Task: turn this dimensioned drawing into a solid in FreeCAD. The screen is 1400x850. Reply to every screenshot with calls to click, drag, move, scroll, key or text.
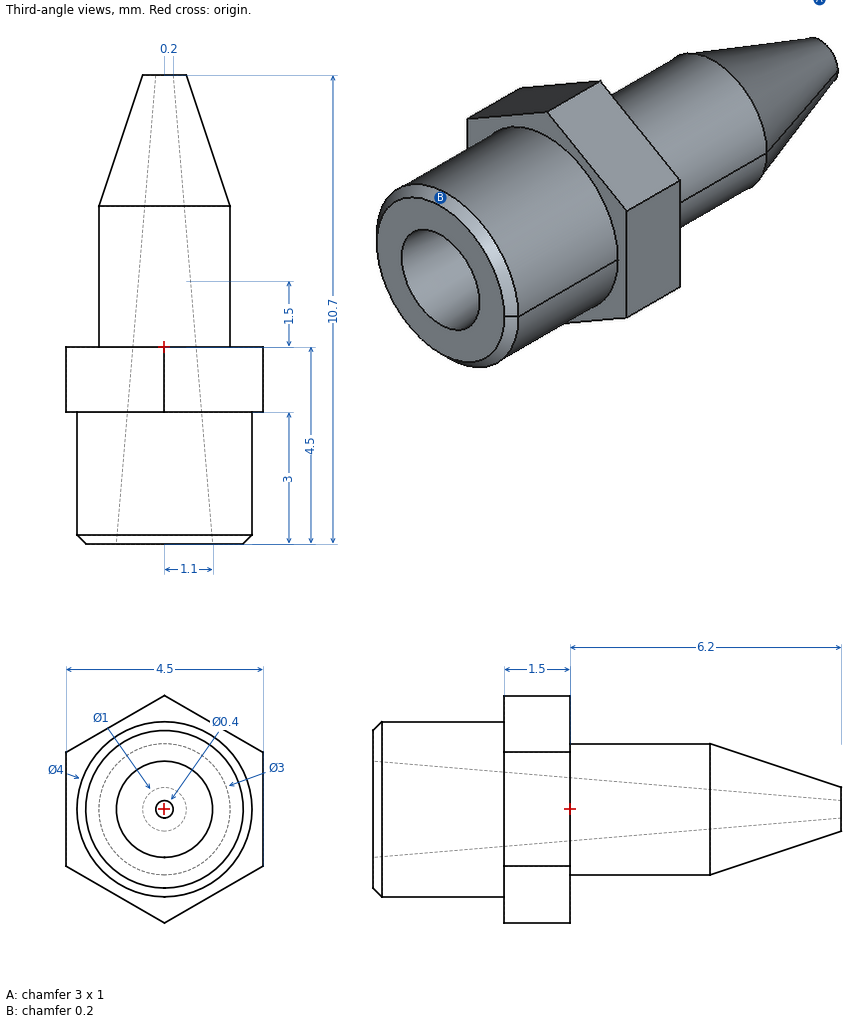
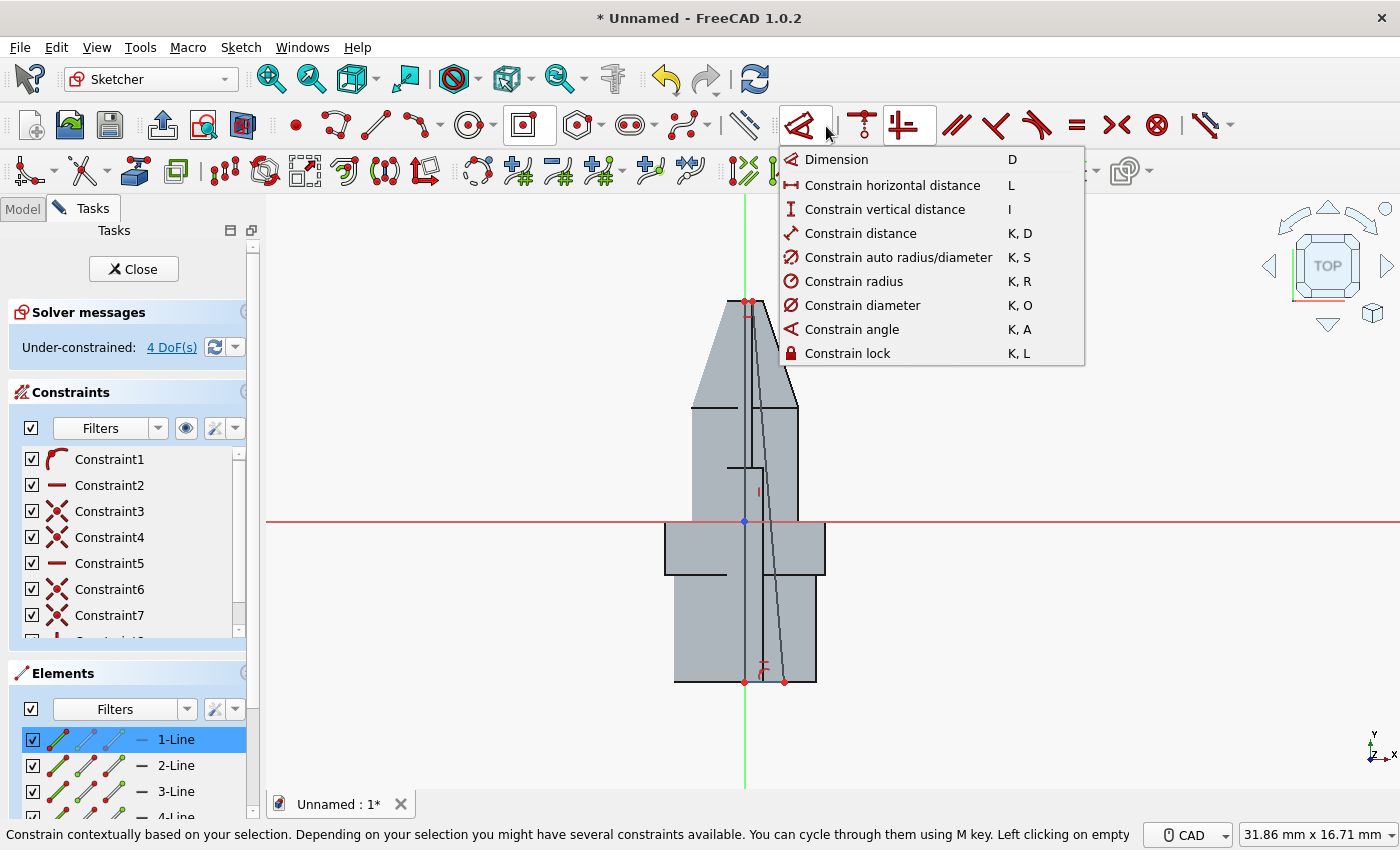
click(932, 185)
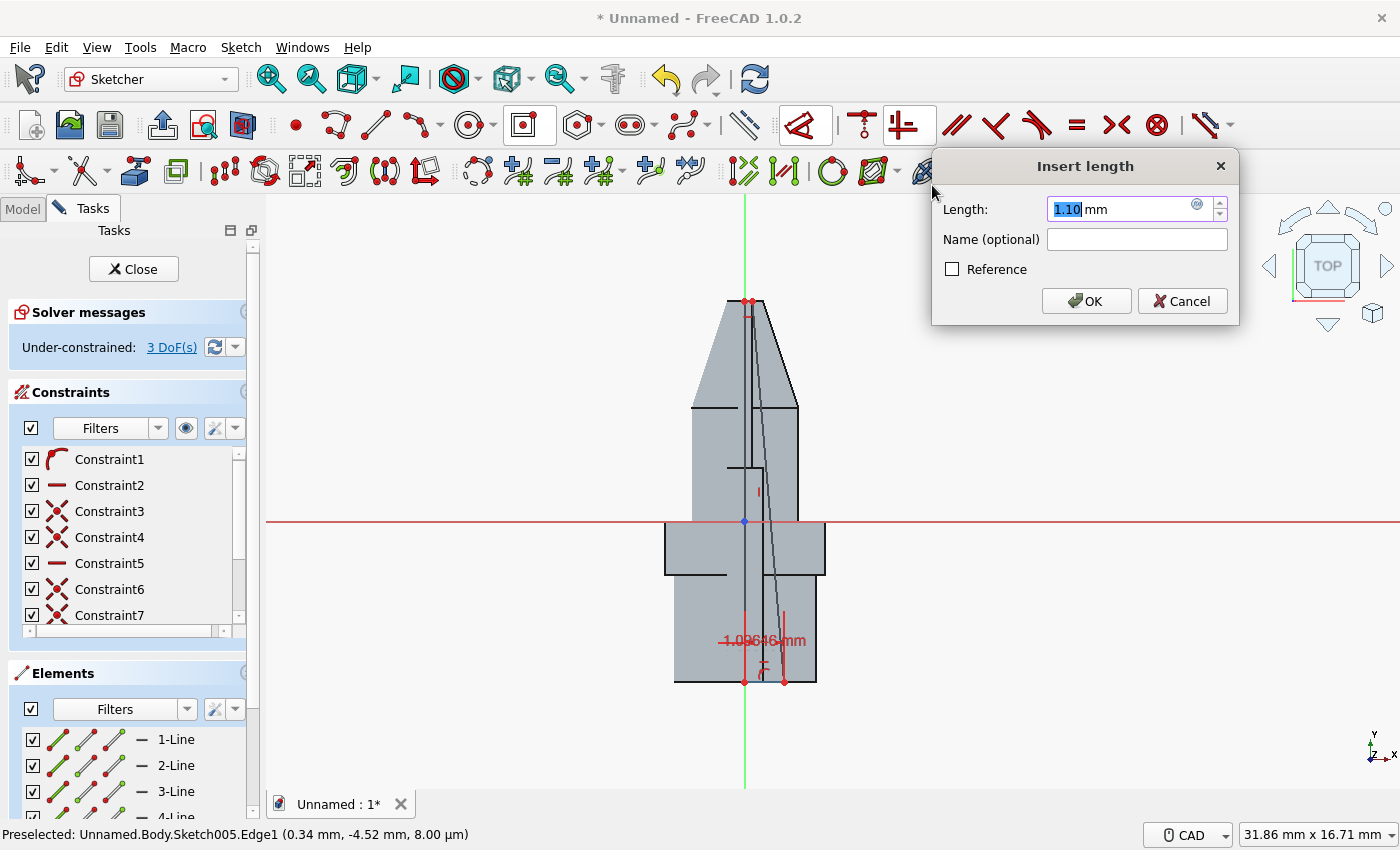
text(1.1)
key(Return)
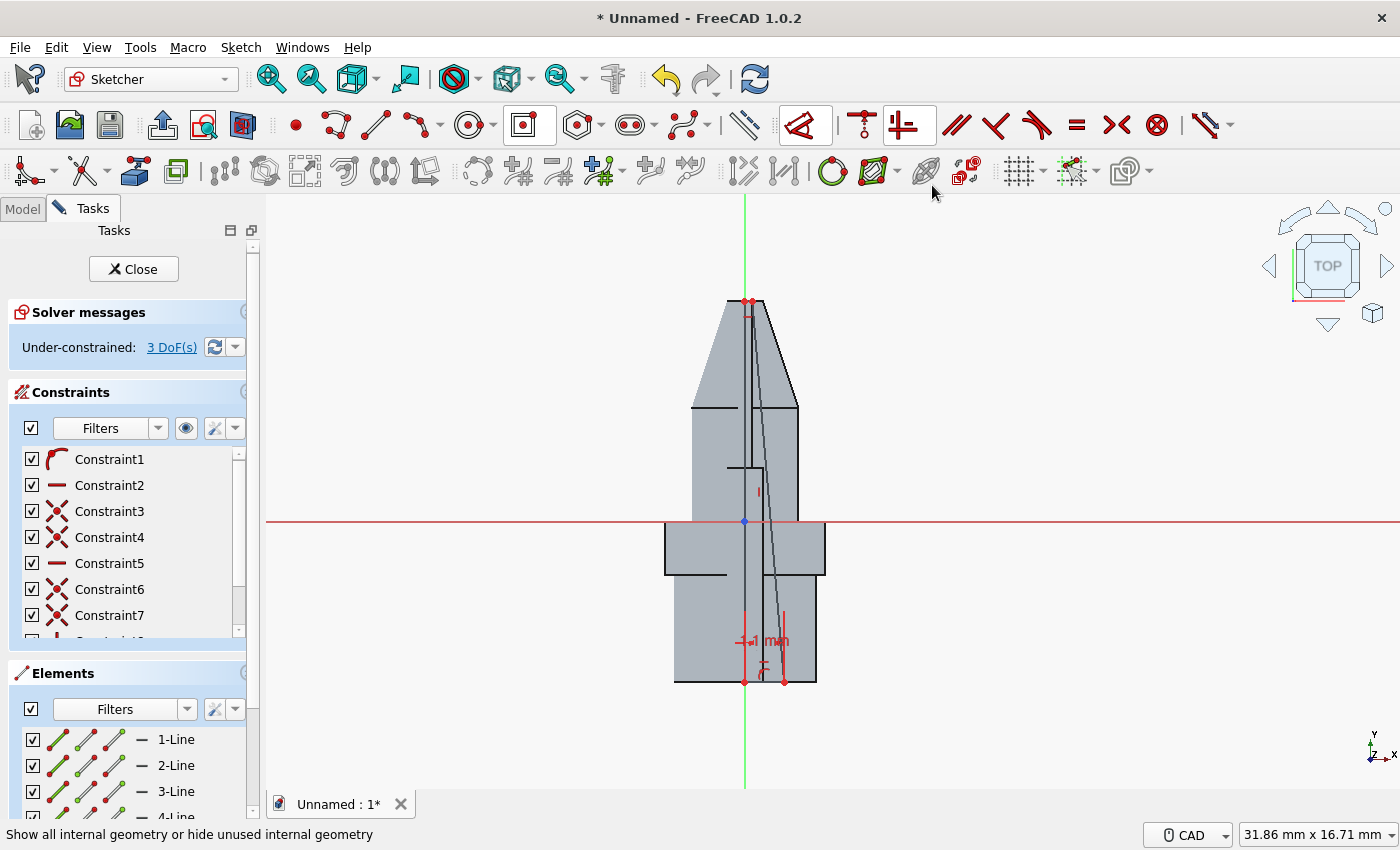
scroll(749, 301, up, 9)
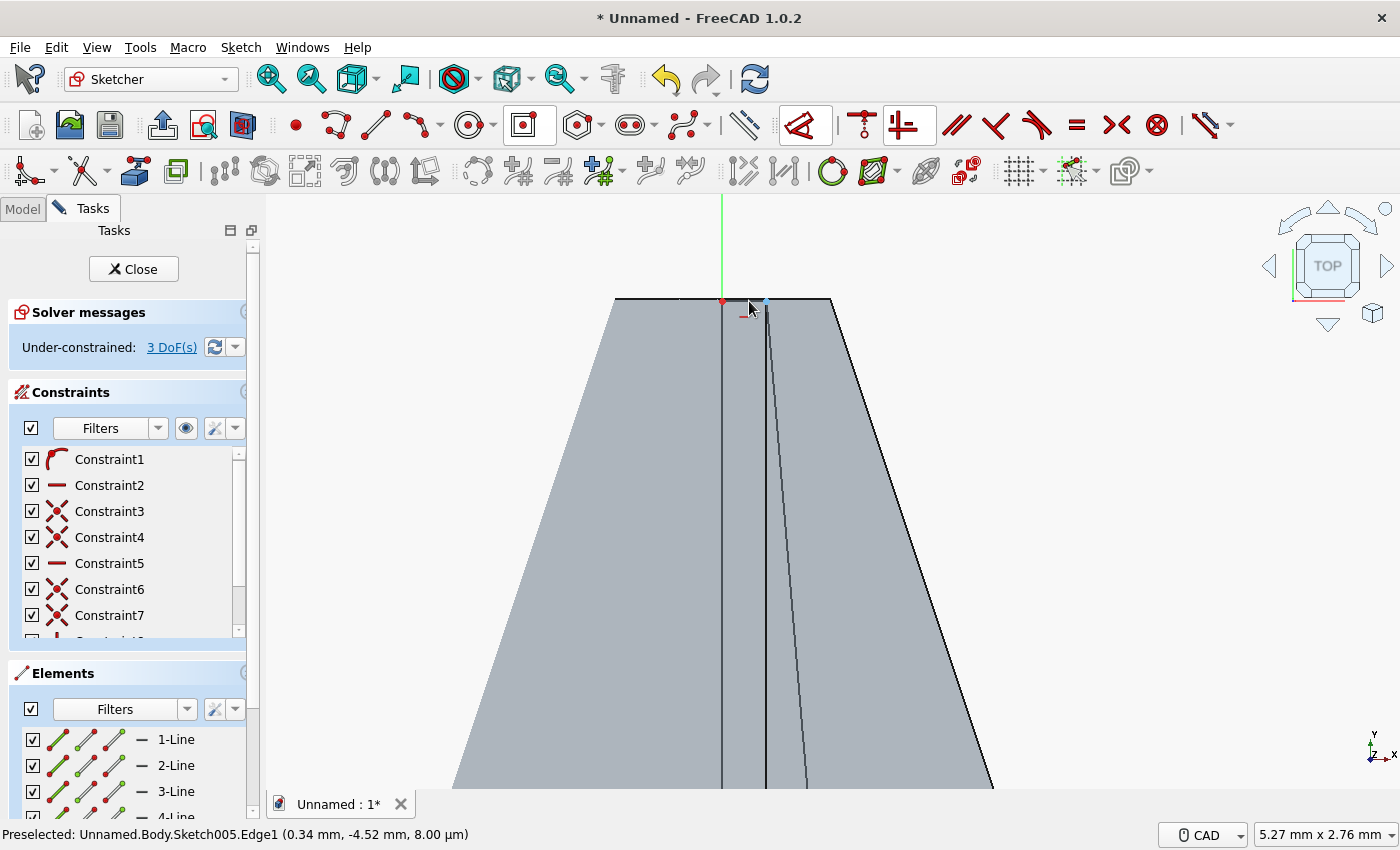
click(745, 301)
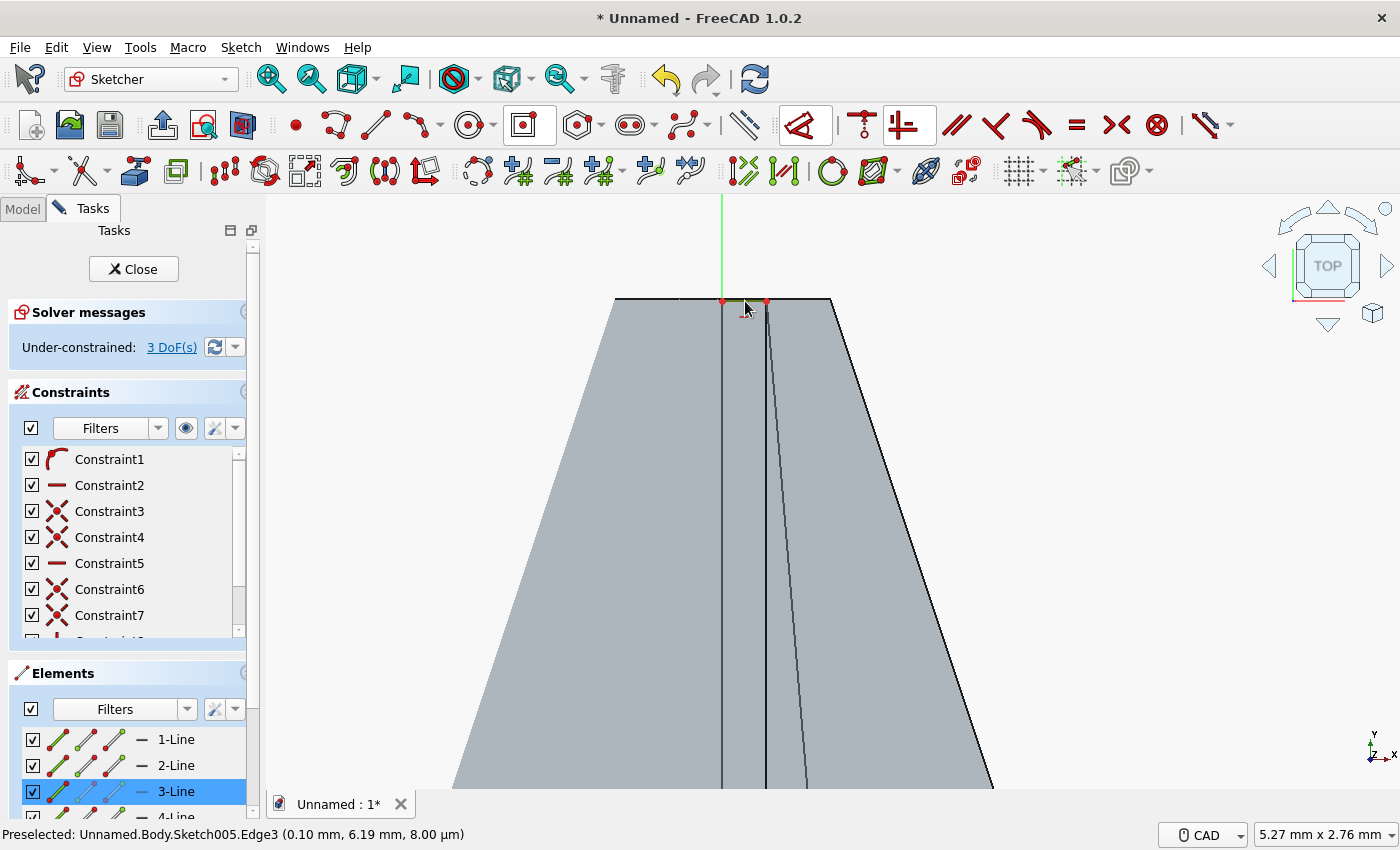
click(826, 126)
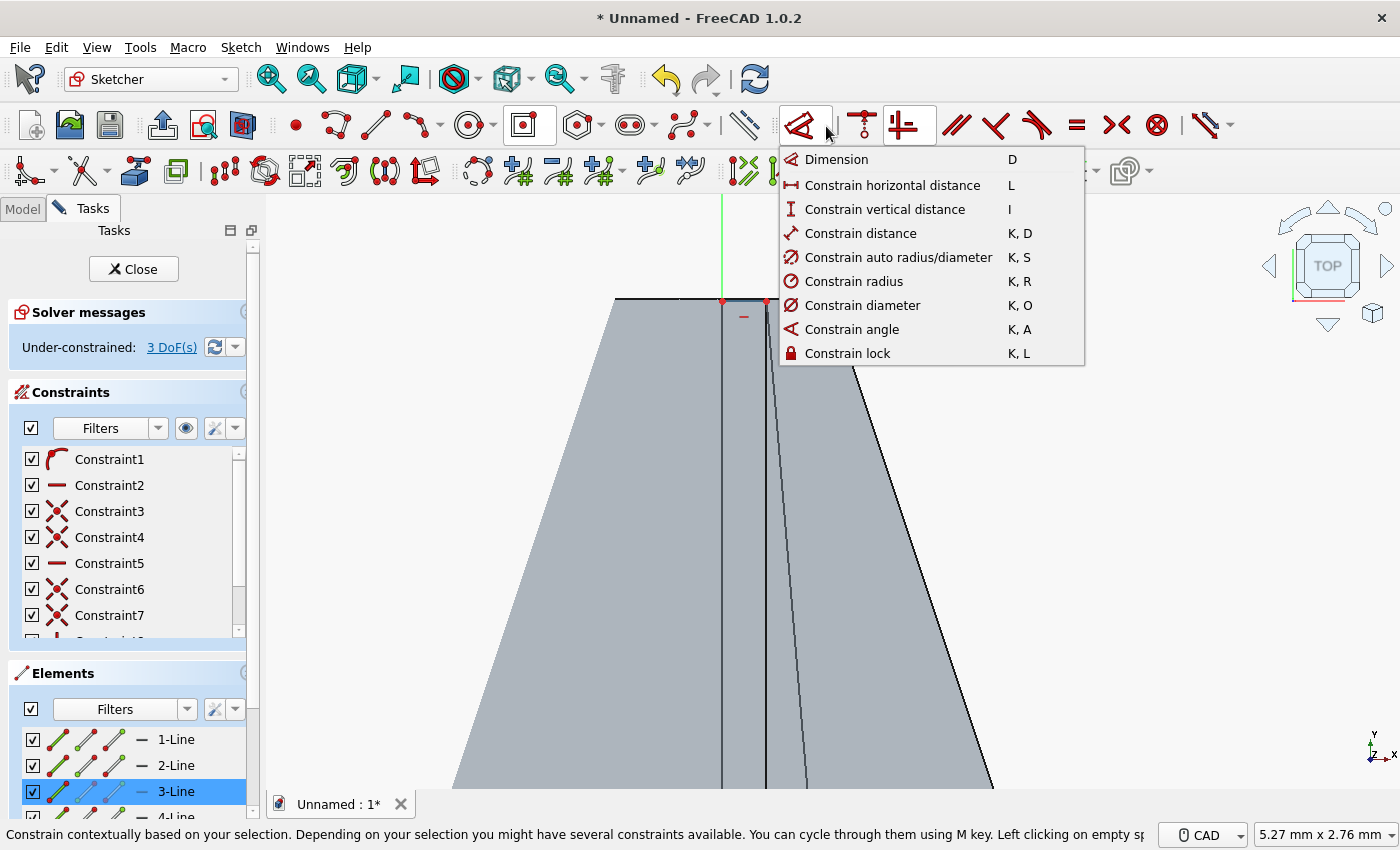
click(932, 185)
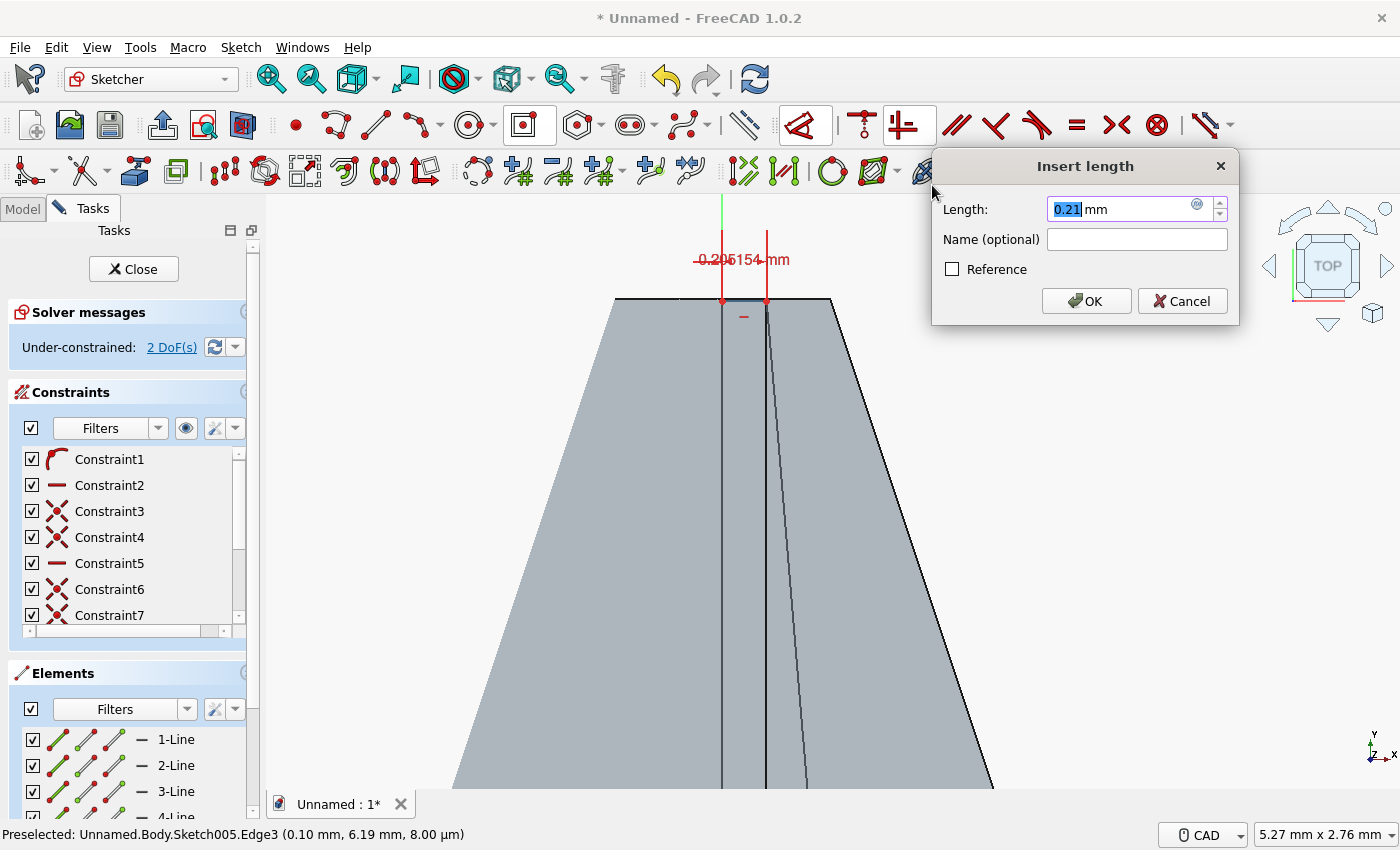
text(0.2)
key(Return)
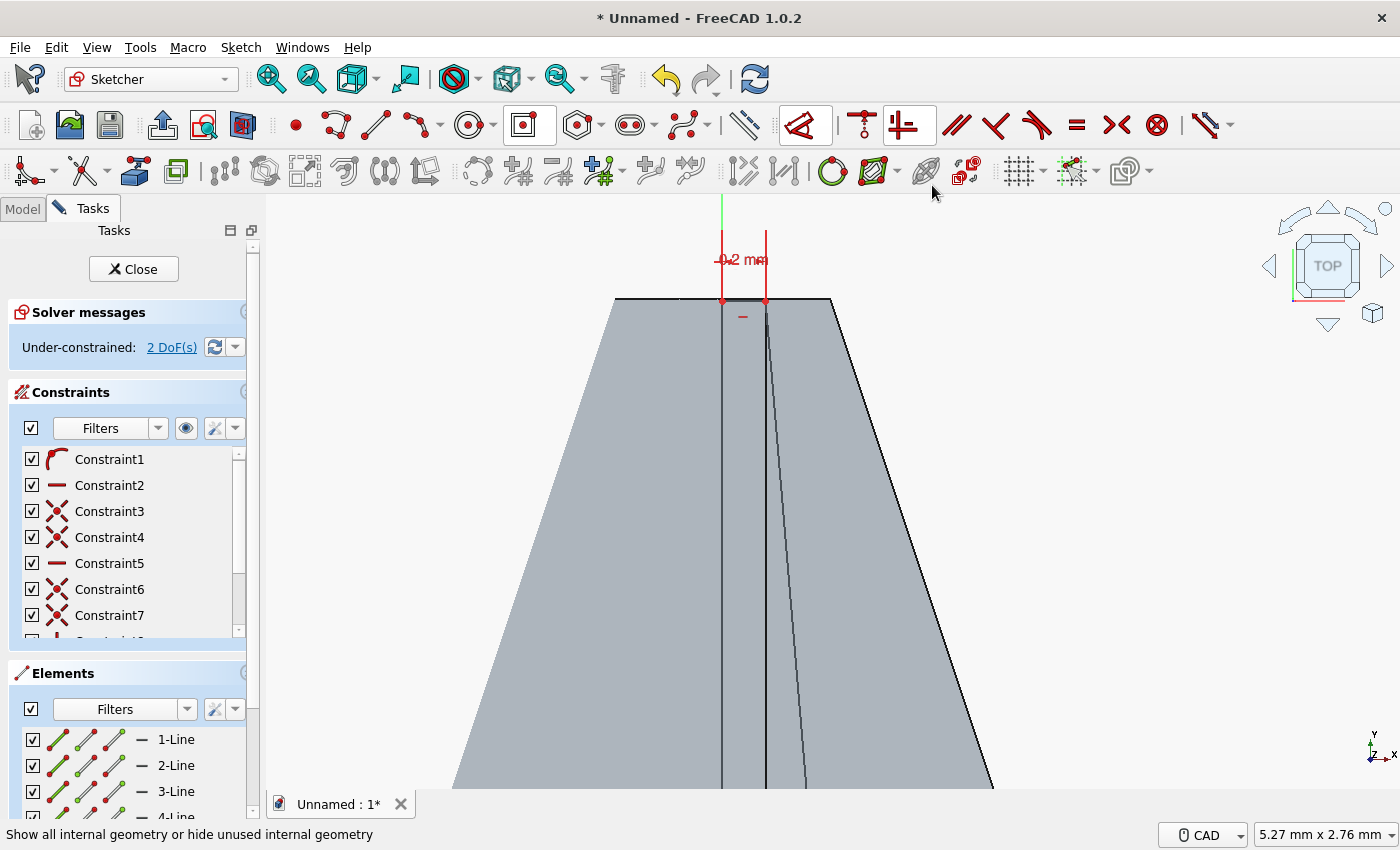
scroll(749, 301, down, 9)